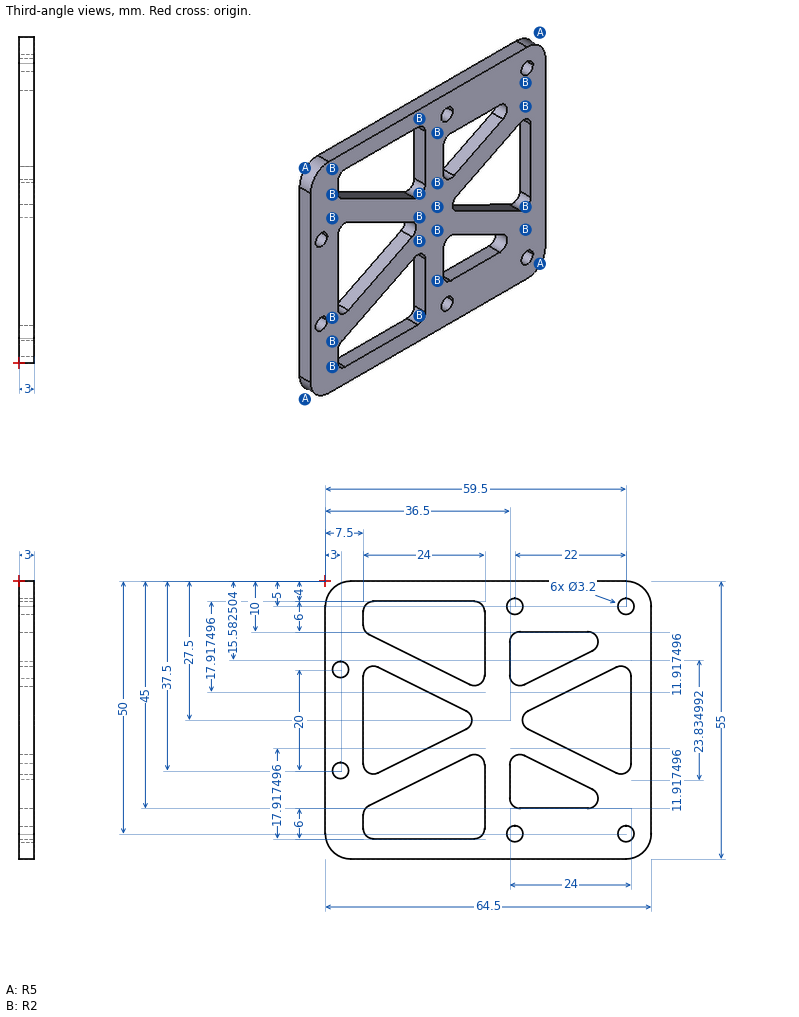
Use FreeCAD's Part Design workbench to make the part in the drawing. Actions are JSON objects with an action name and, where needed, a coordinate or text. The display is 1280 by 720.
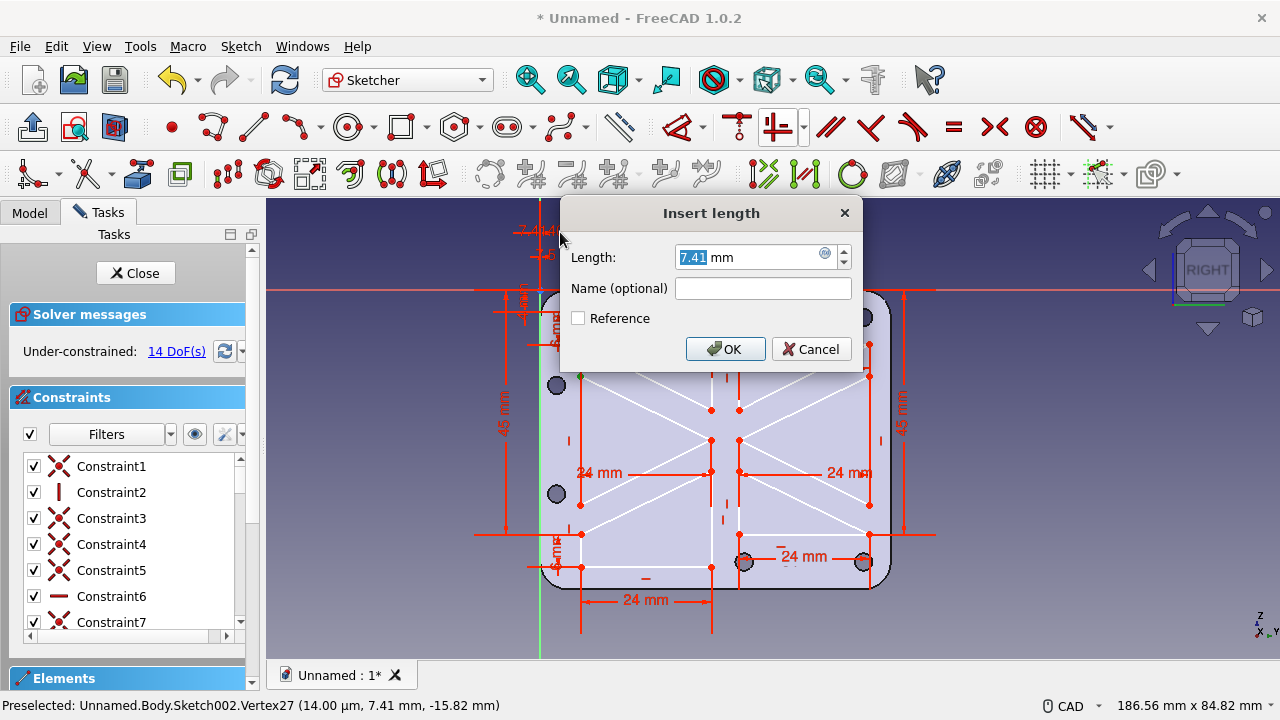
{"action": "type", "text": "7.5"}
{"action": "key", "text": "Return"}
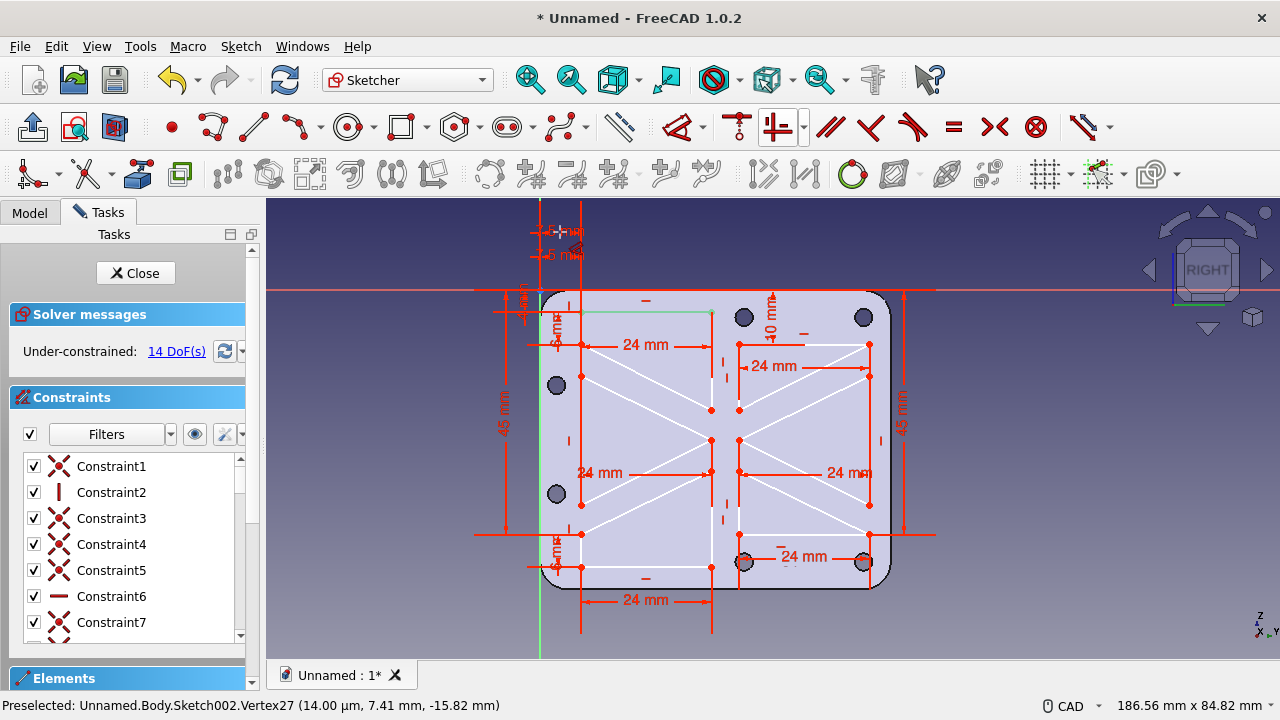
{"action": "left_click", "coordinate": [581, 535]}
{"action": "left_click", "coordinate": [561, 593]}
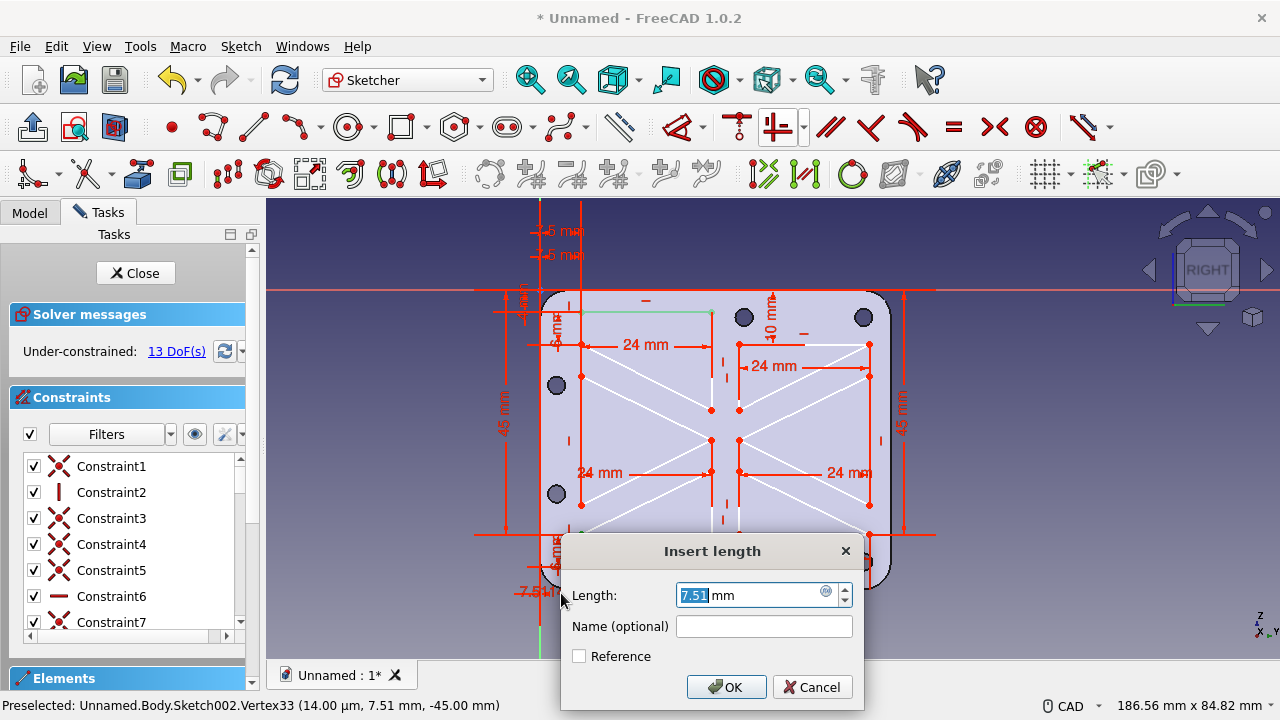
{"action": "type", "text": "7.5"}
{"action": "key", "text": "Return"}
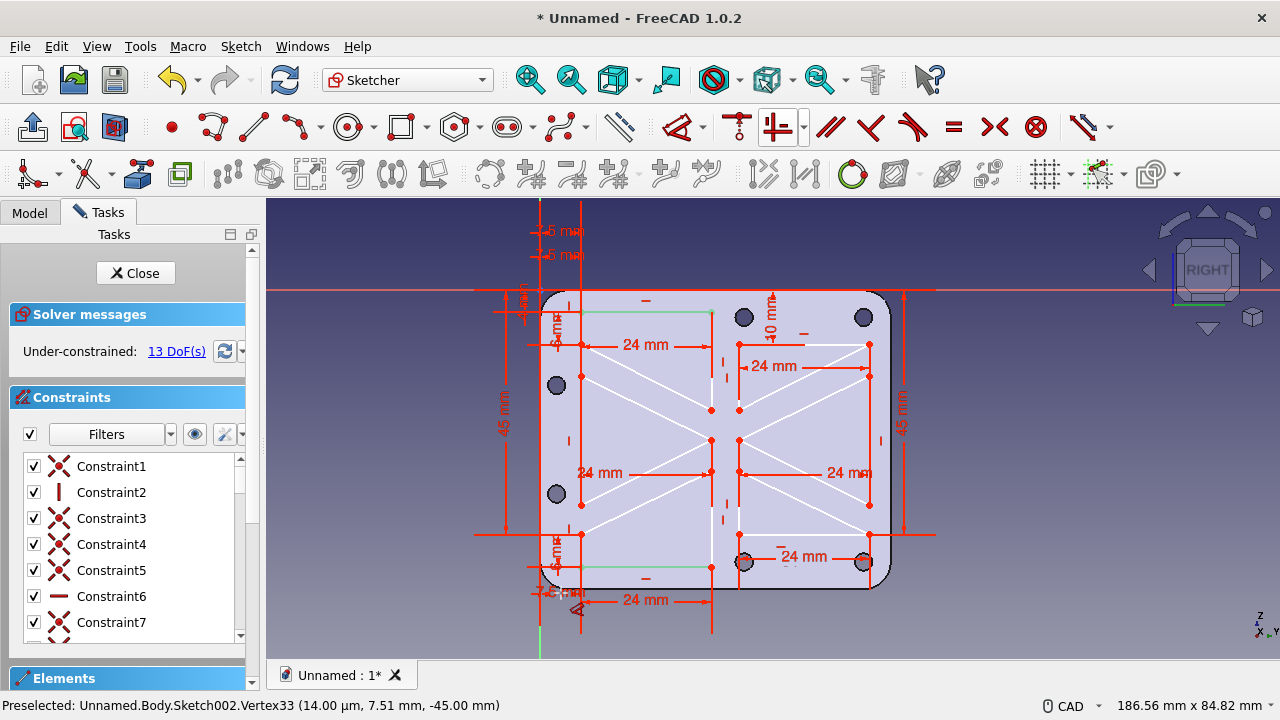
{"action": "left_click", "coordinate": [739, 440]}
{"action": "left_click", "coordinate": [640, 256]}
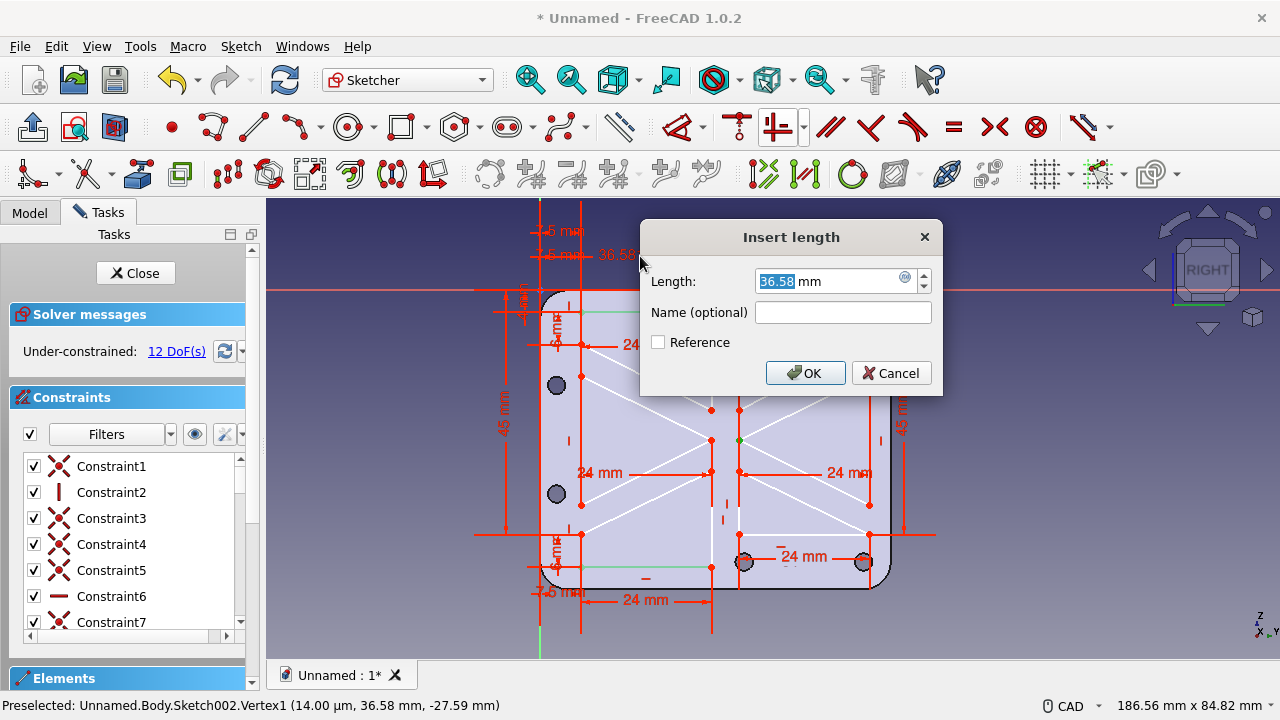
{"action": "type", "text": "36.5"}
{"action": "key", "text": "Return"}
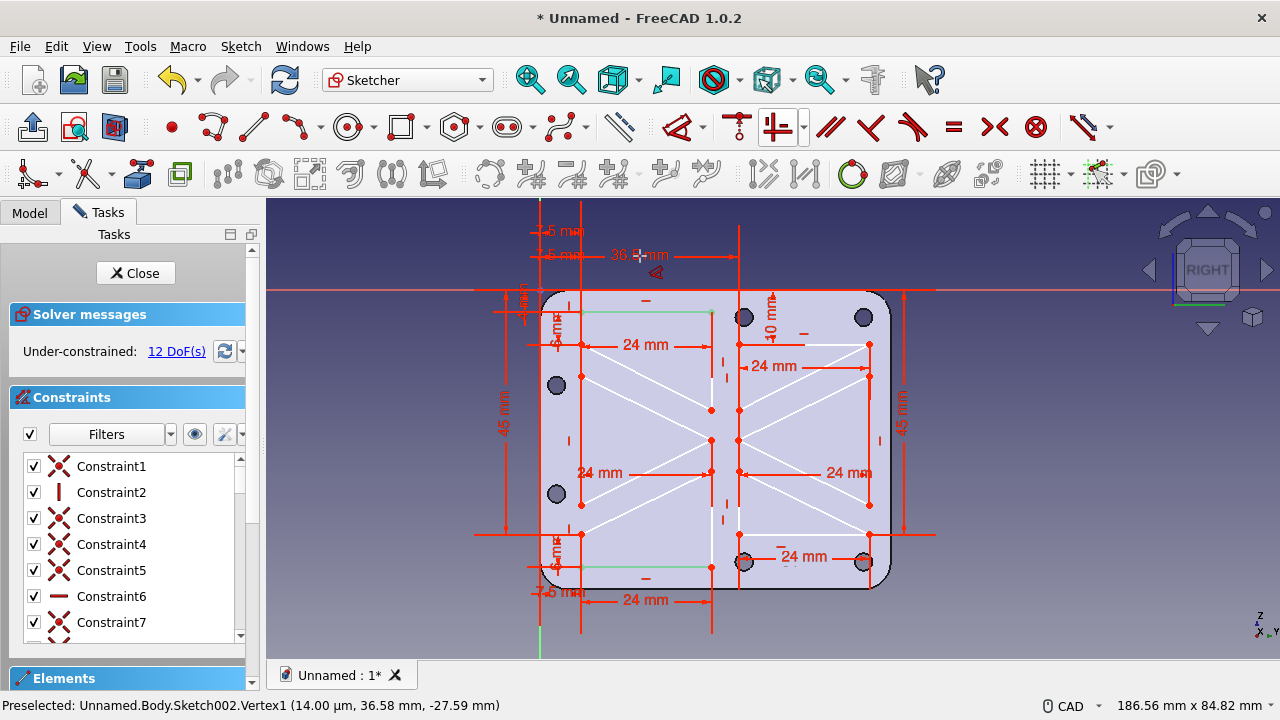
{"action": "left_click", "coordinate": [739, 440]}
{"action": "left_click", "coordinate": [506, 365]}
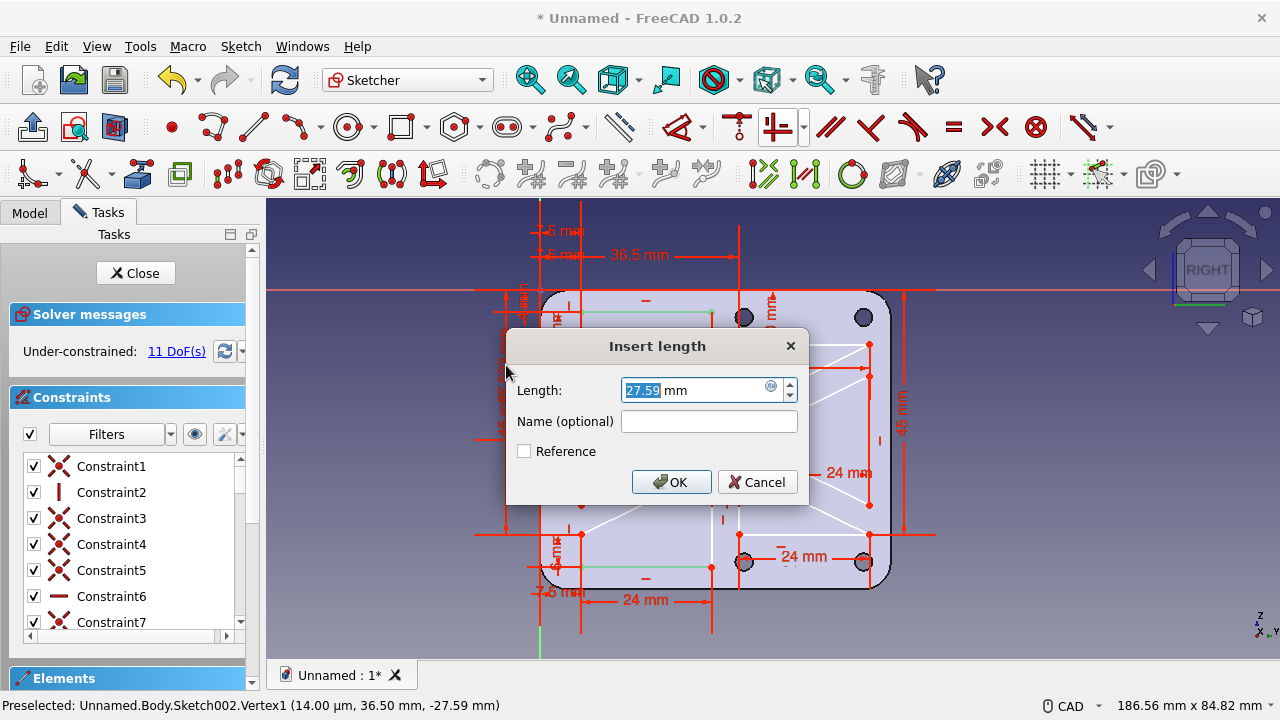
{"action": "type", "text": "27.5"}
{"action": "key", "text": "Return"}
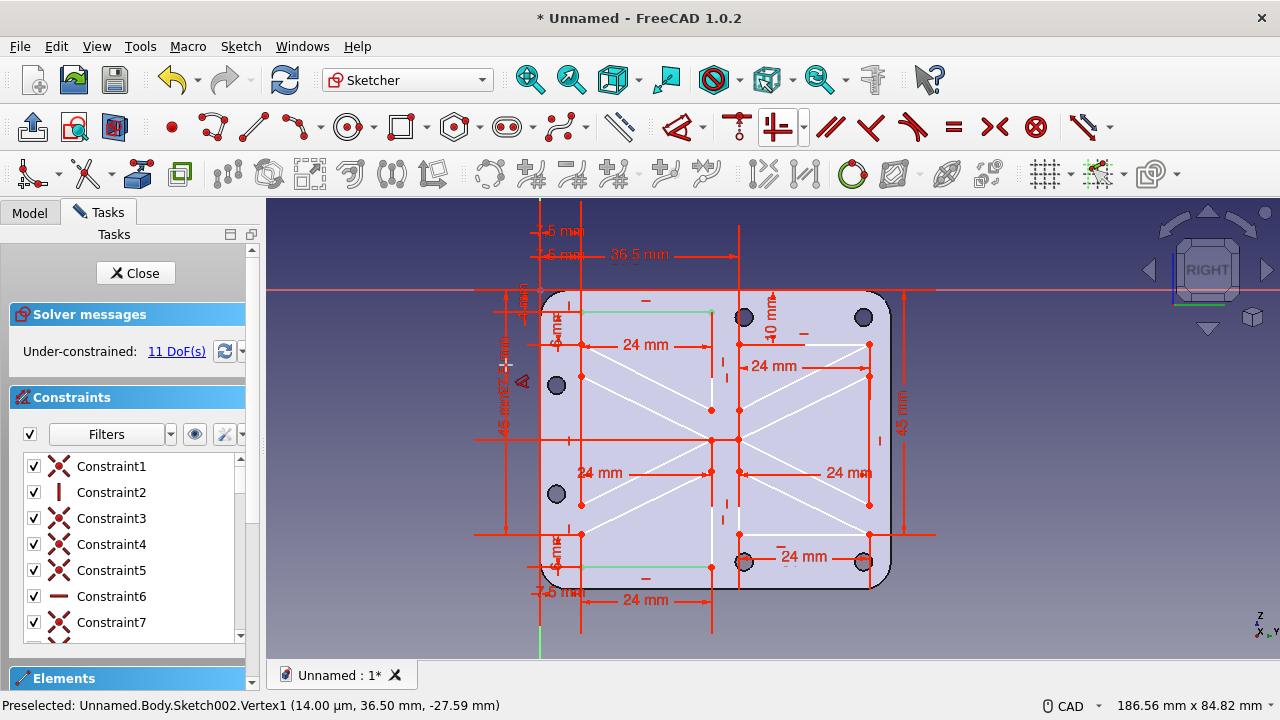
{"action": "left_click", "coordinate": [739, 471]}
{"action": "left_click", "coordinate": [685, 505]}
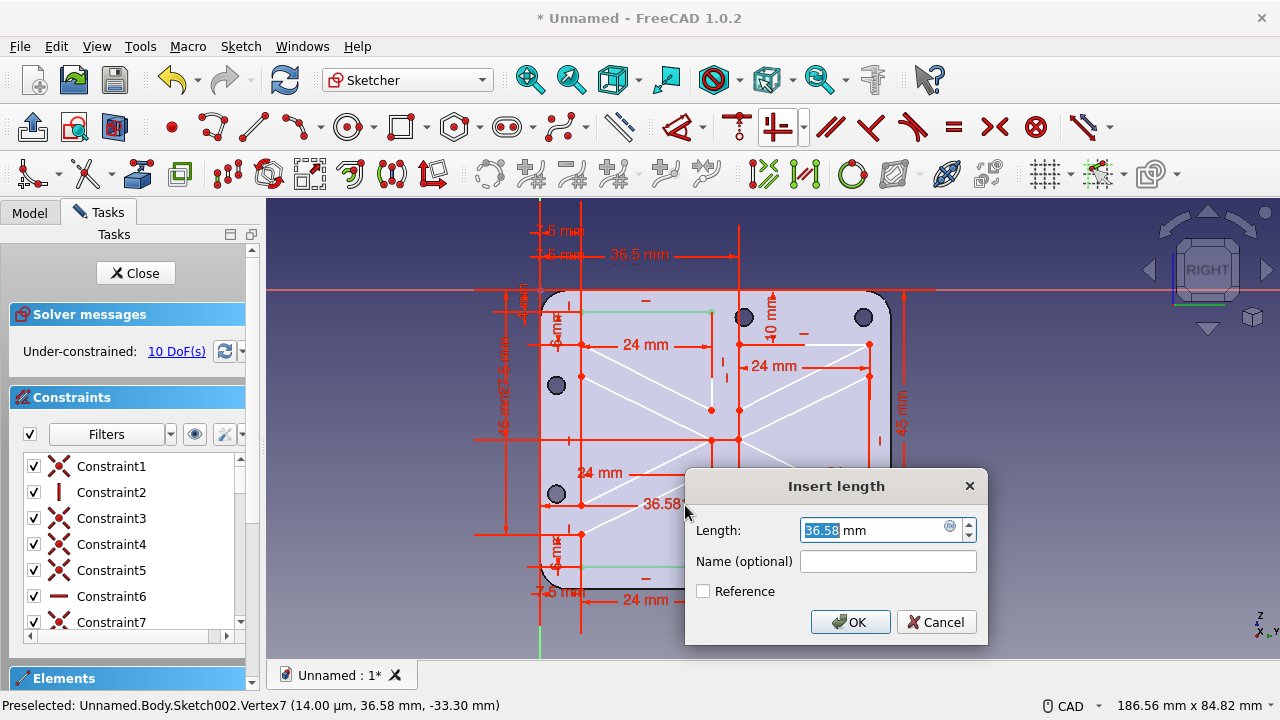
{"action": "type", "text": "36.5"}
{"action": "key", "text": "Return"}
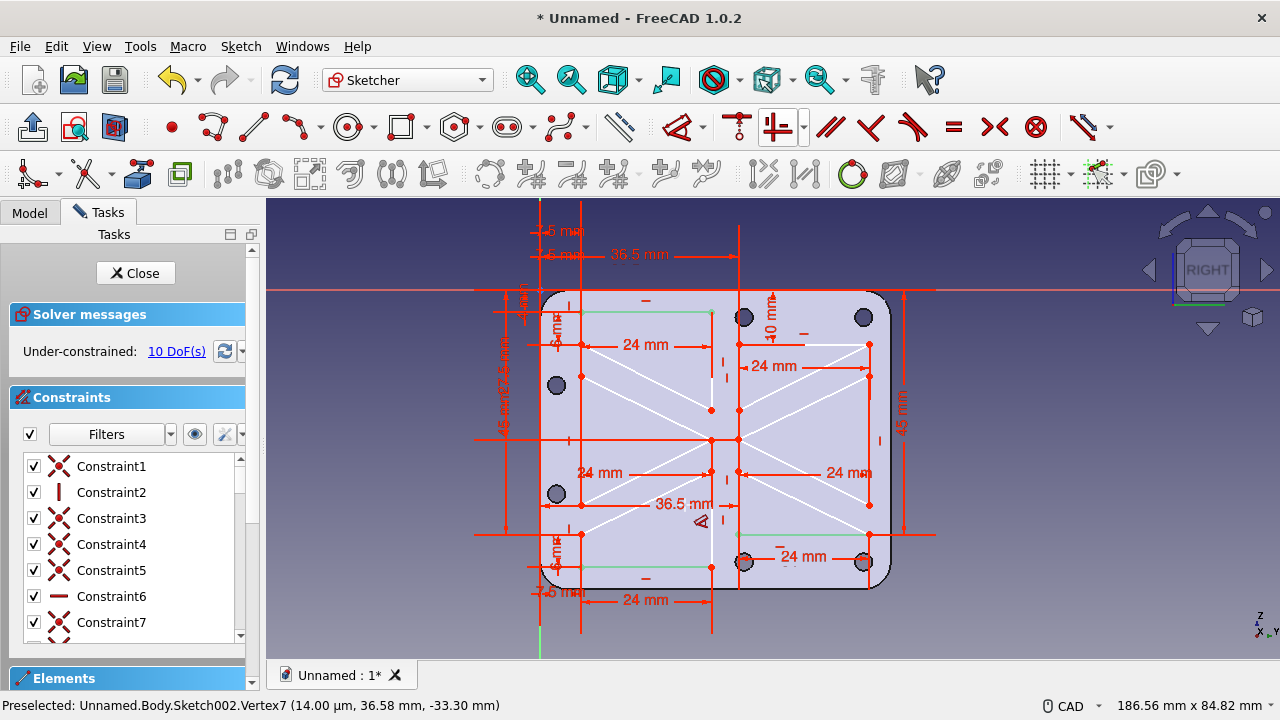
{"action": "left_click", "coordinate": [739, 345]}
{"action": "left_click", "coordinate": [685, 379]}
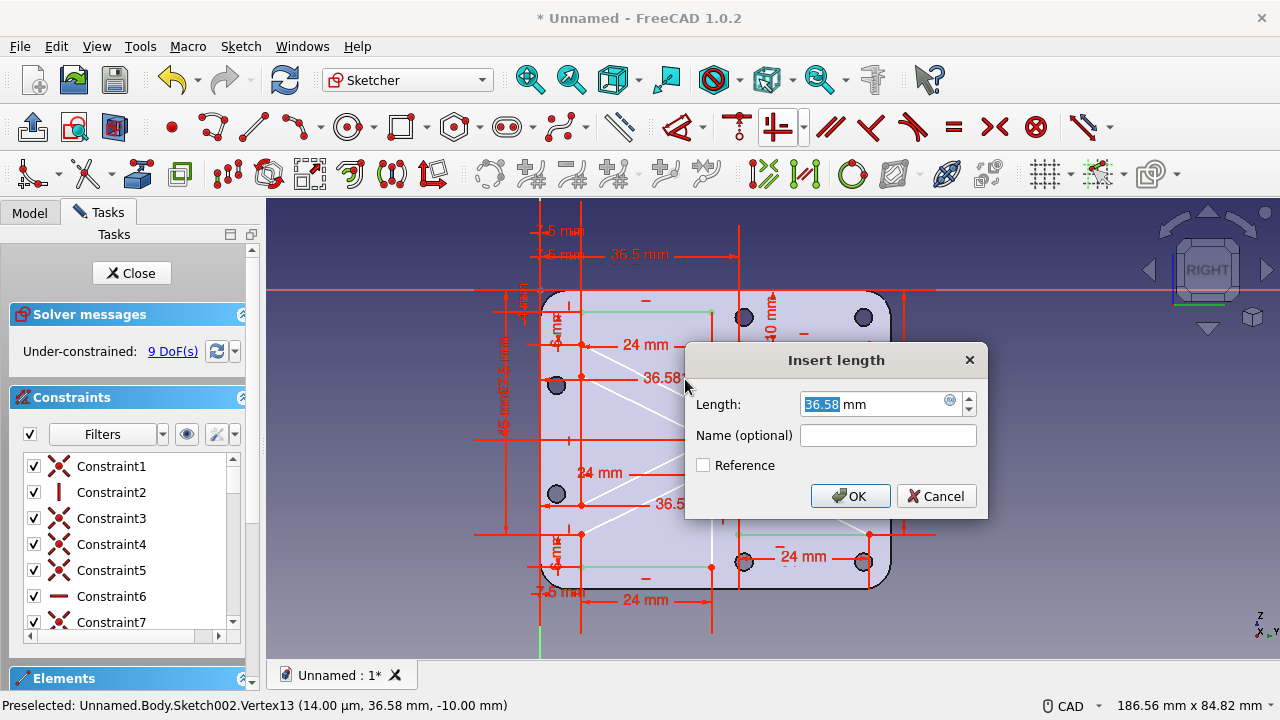
{"action": "type", "text": "36.5"}
{"action": "key", "text": "Return"}